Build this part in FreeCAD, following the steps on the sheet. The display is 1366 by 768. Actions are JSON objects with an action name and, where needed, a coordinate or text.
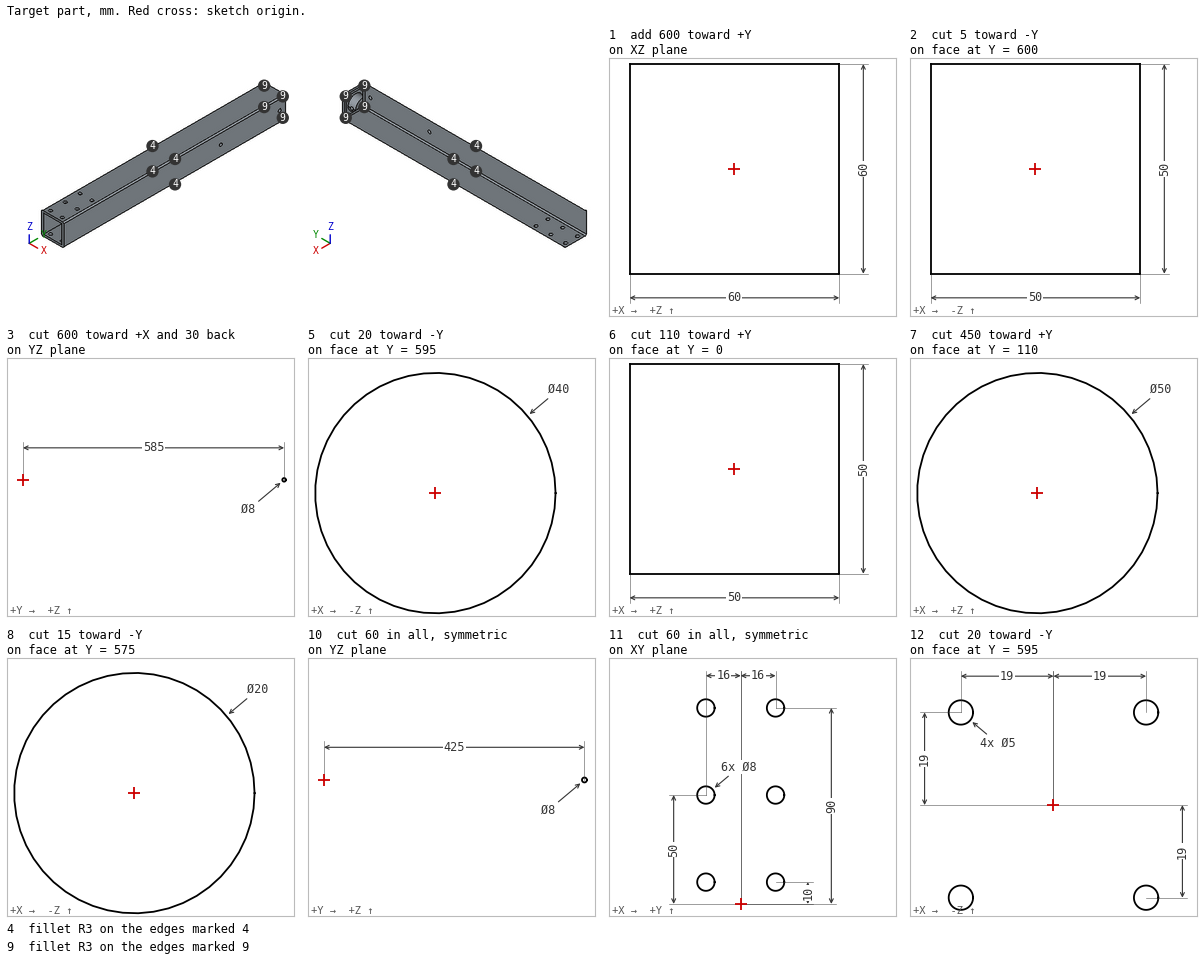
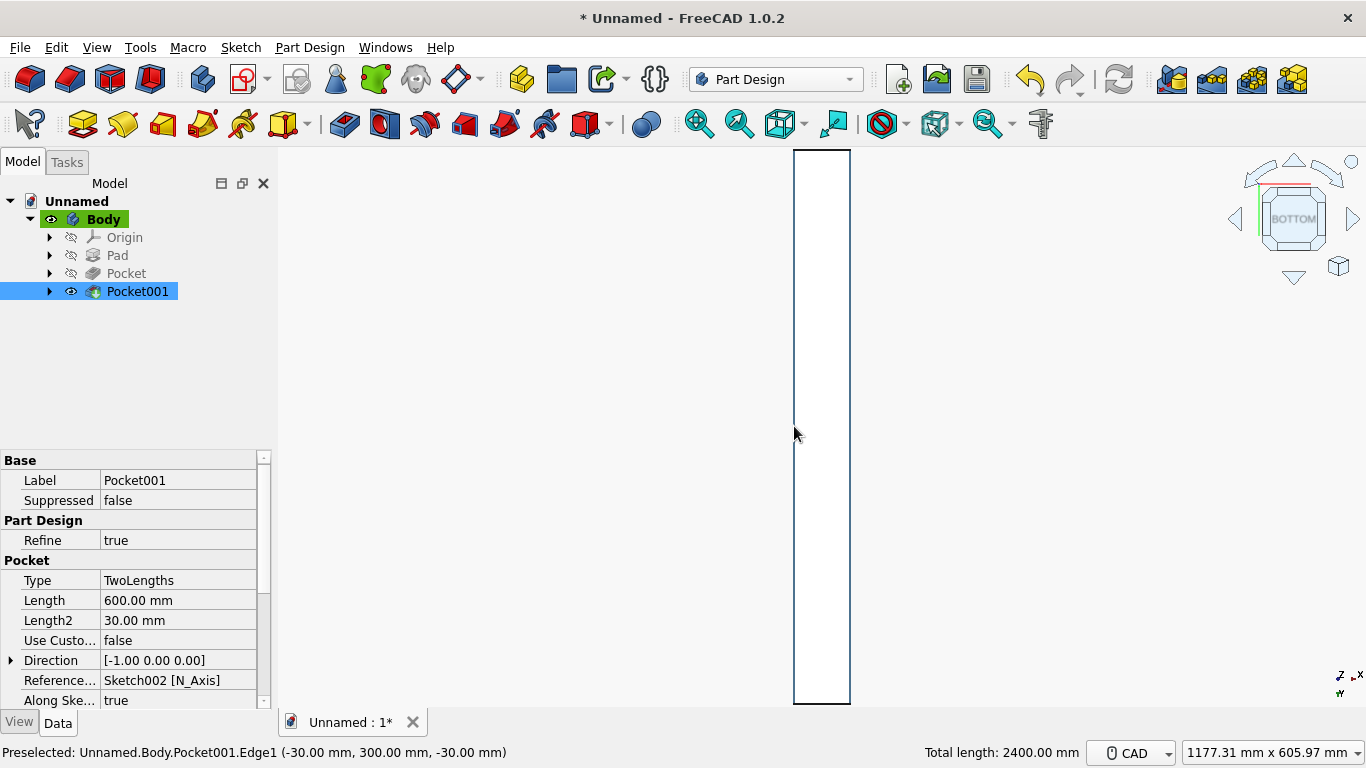
{"action": "left_click", "coordinate": [30, 80]}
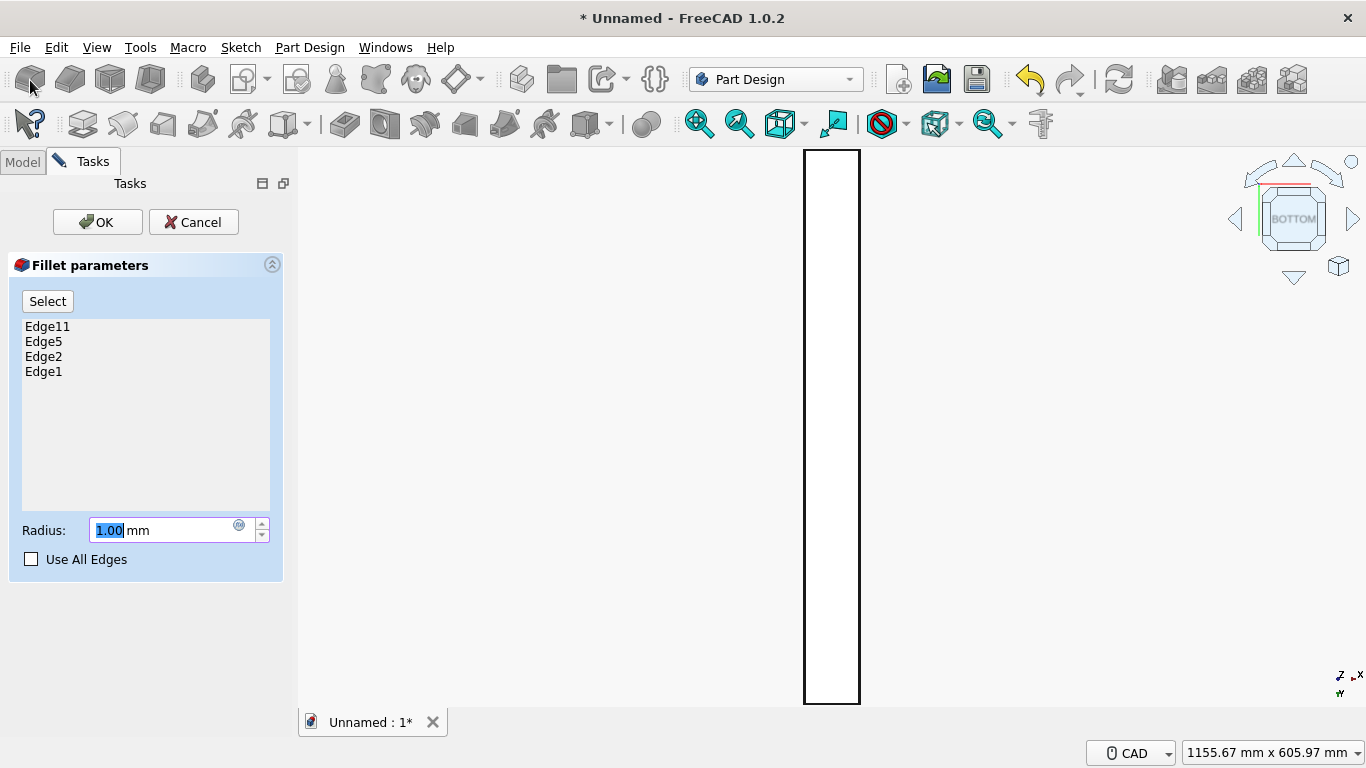
{"action": "type", "text": "3"}
{"action": "key", "text": "Tab"}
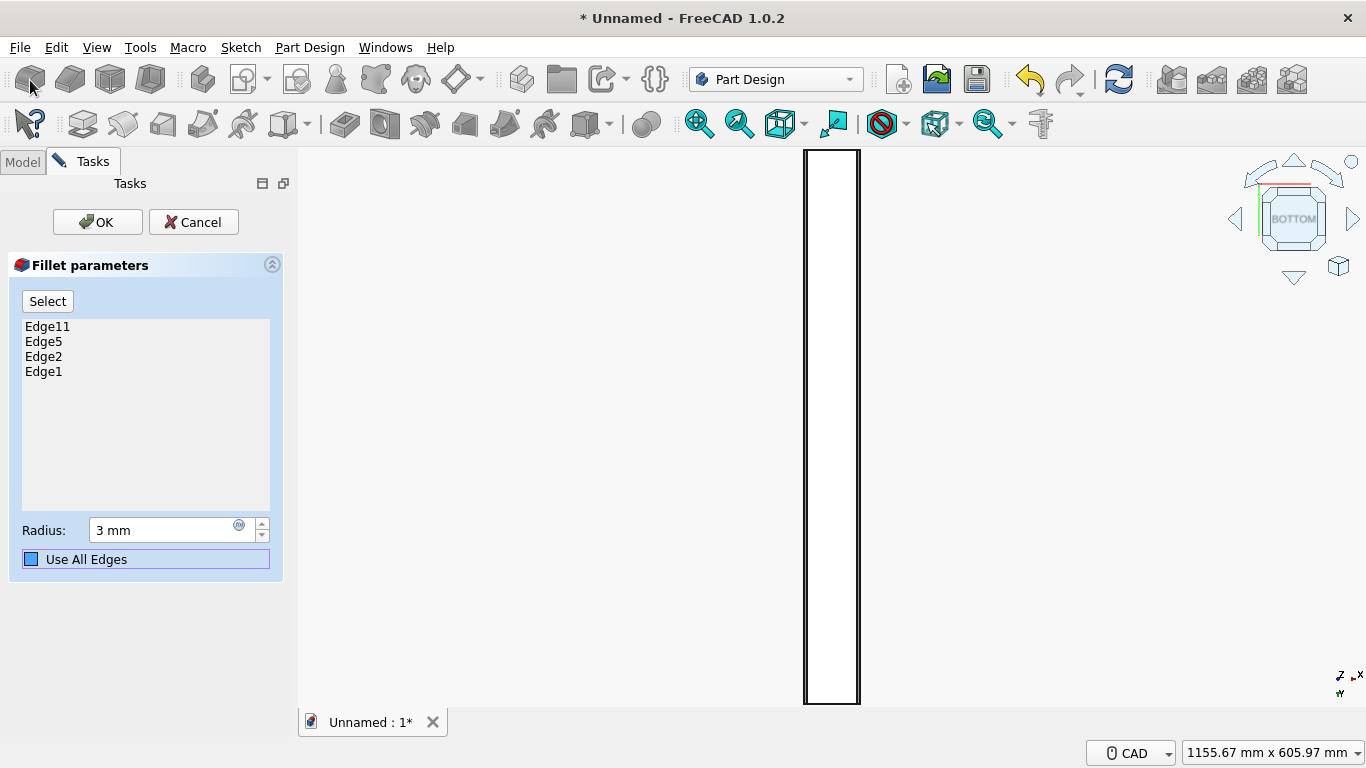
{"action": "left_click", "coordinate": [98, 222]}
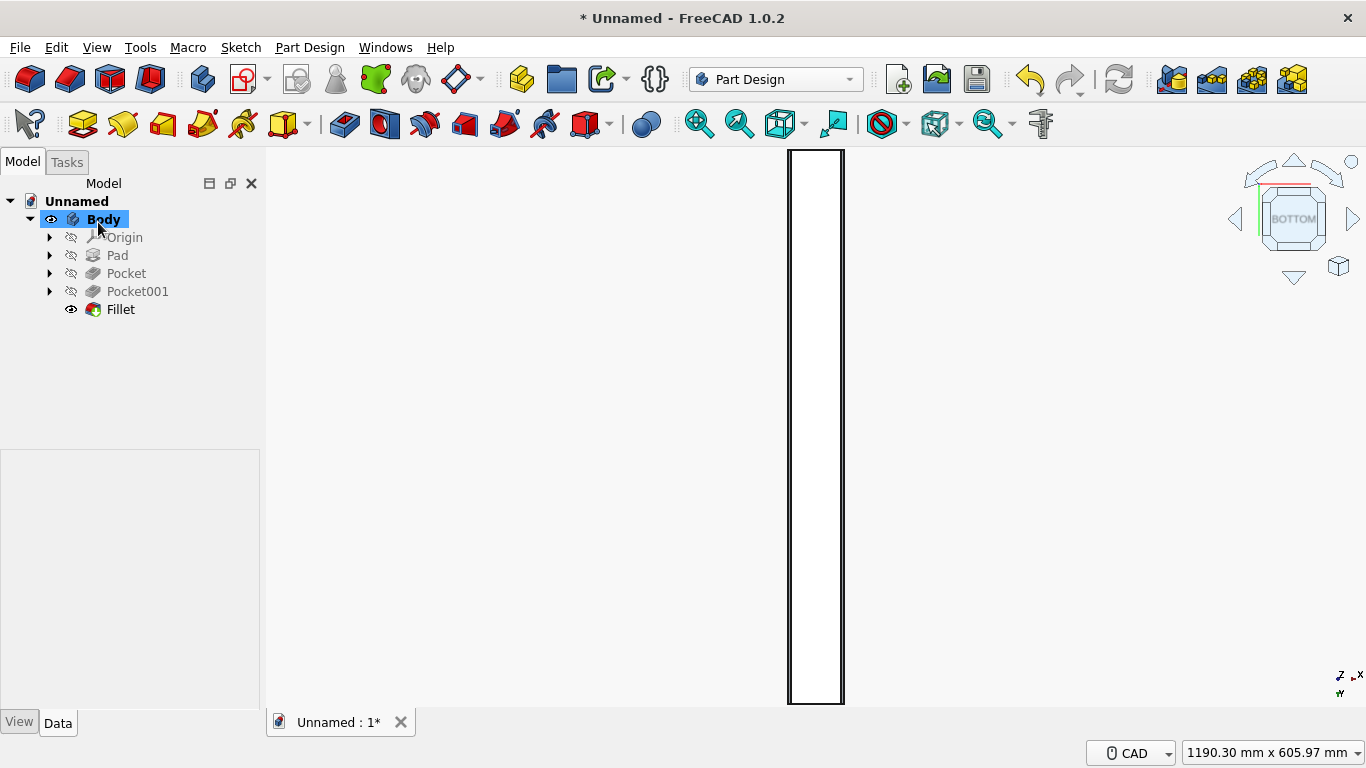
{"action": "key", "text": "4"}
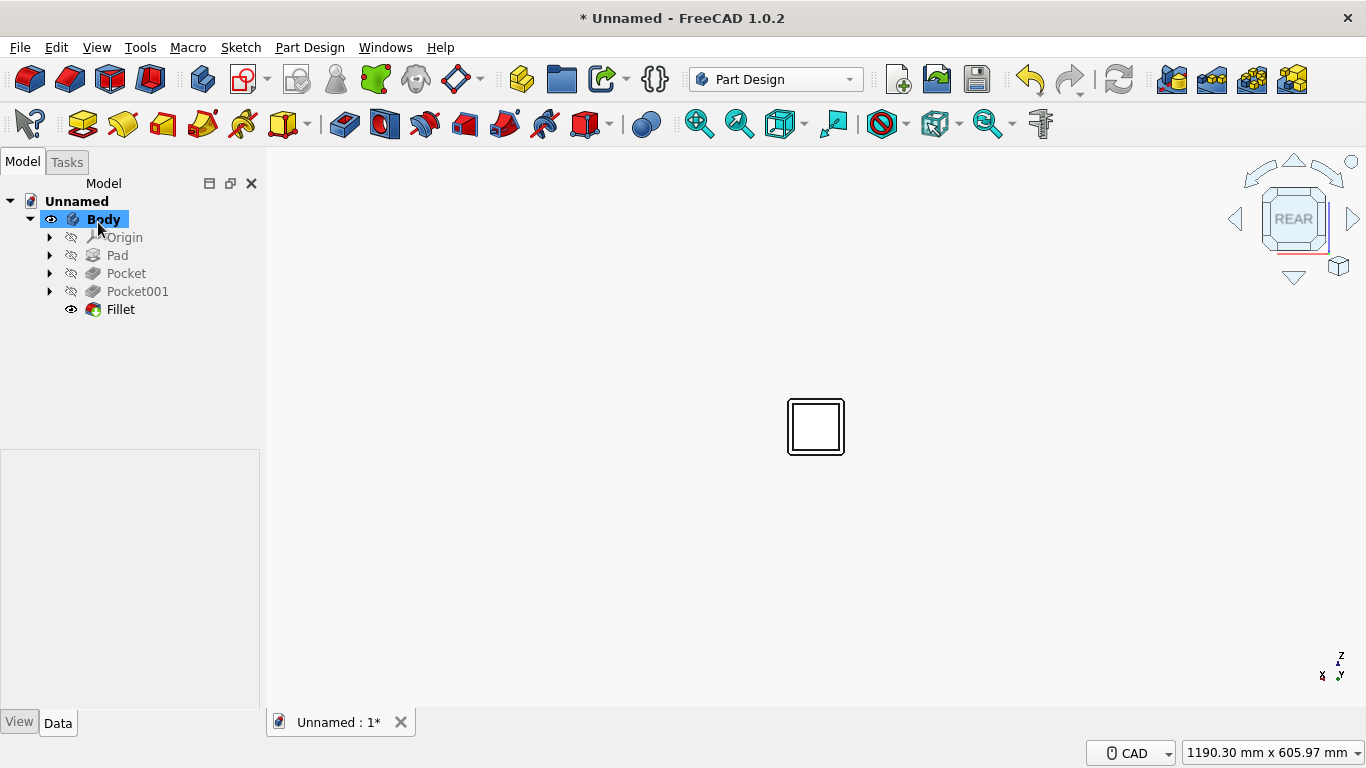
{"action": "left_click", "coordinate": [700, 124]}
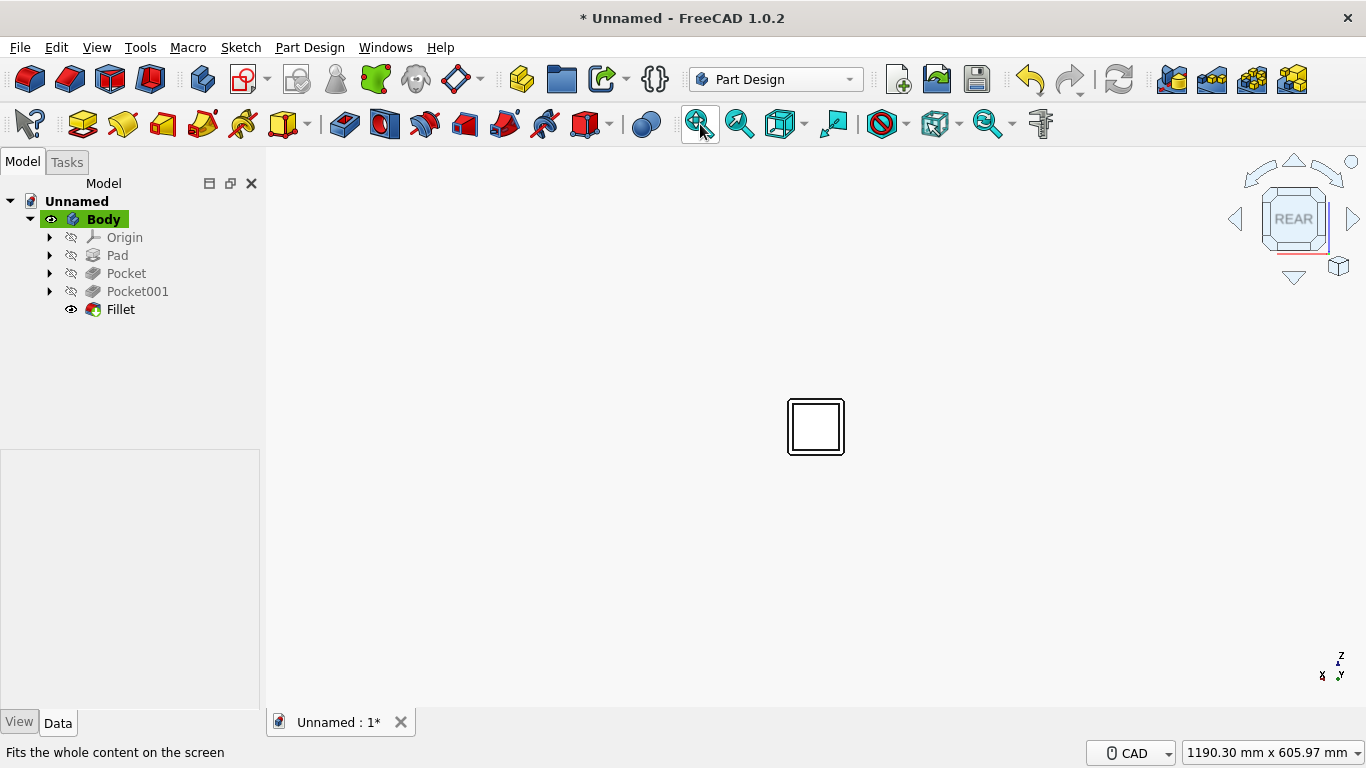
{"action": "left_click", "coordinate": [816, 426]}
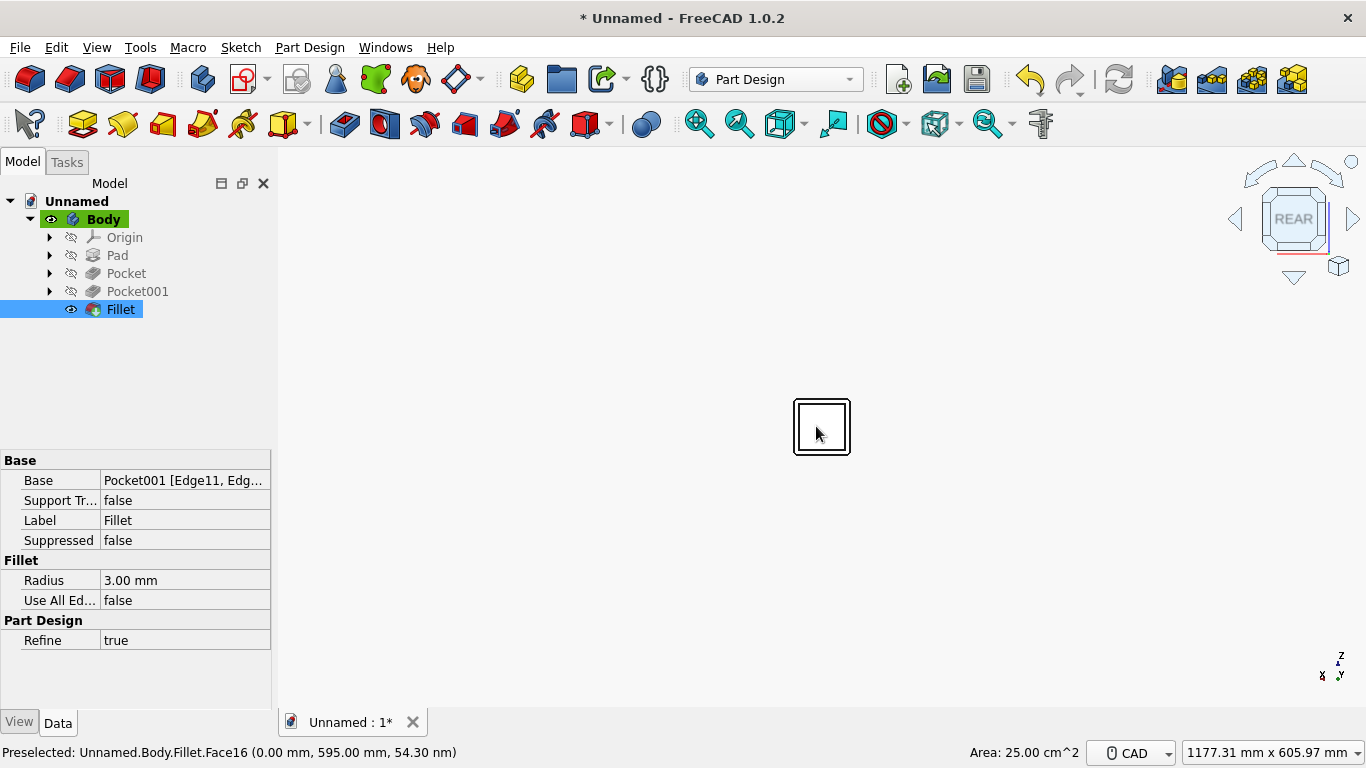
{"action": "left_click", "coordinate": [244, 80]}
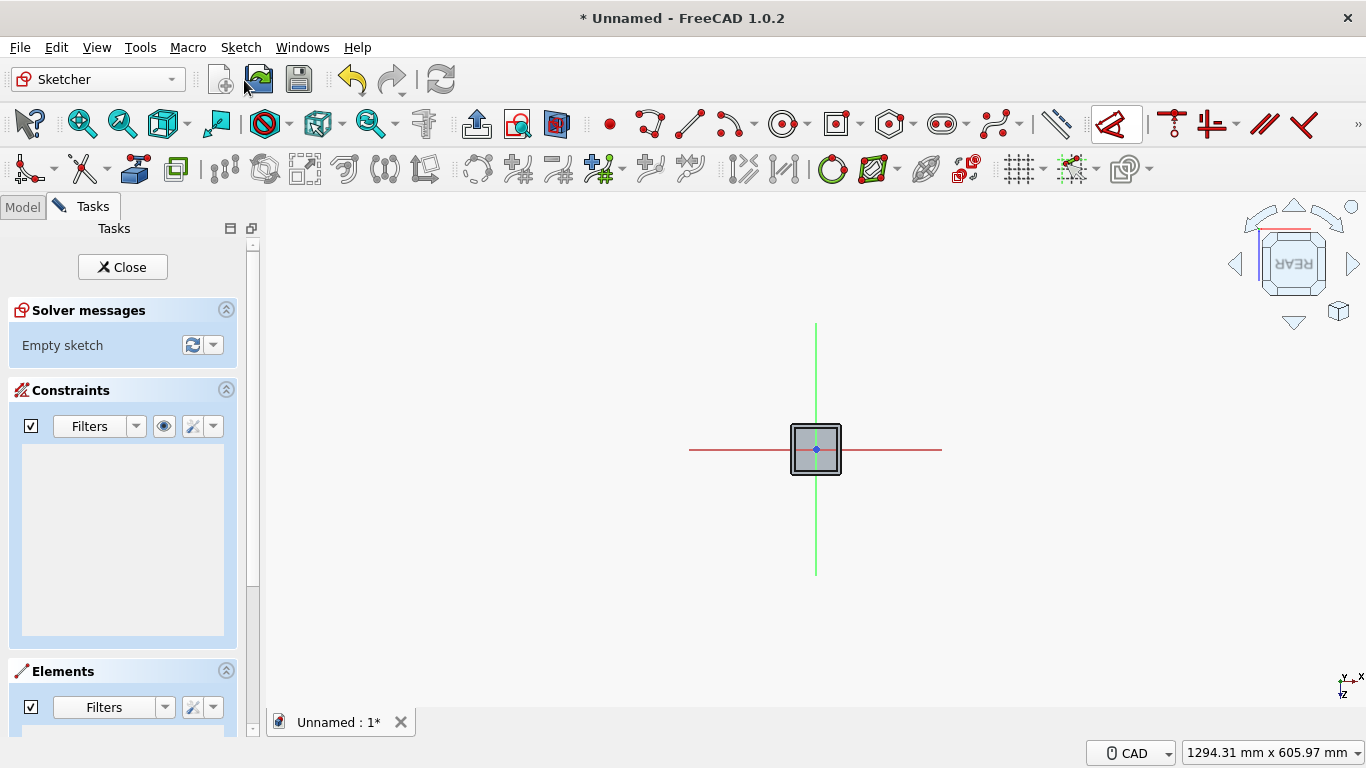
{"action": "scroll", "coordinate": [825, 449], "scroll_direction": "up", "scroll_amount": 11}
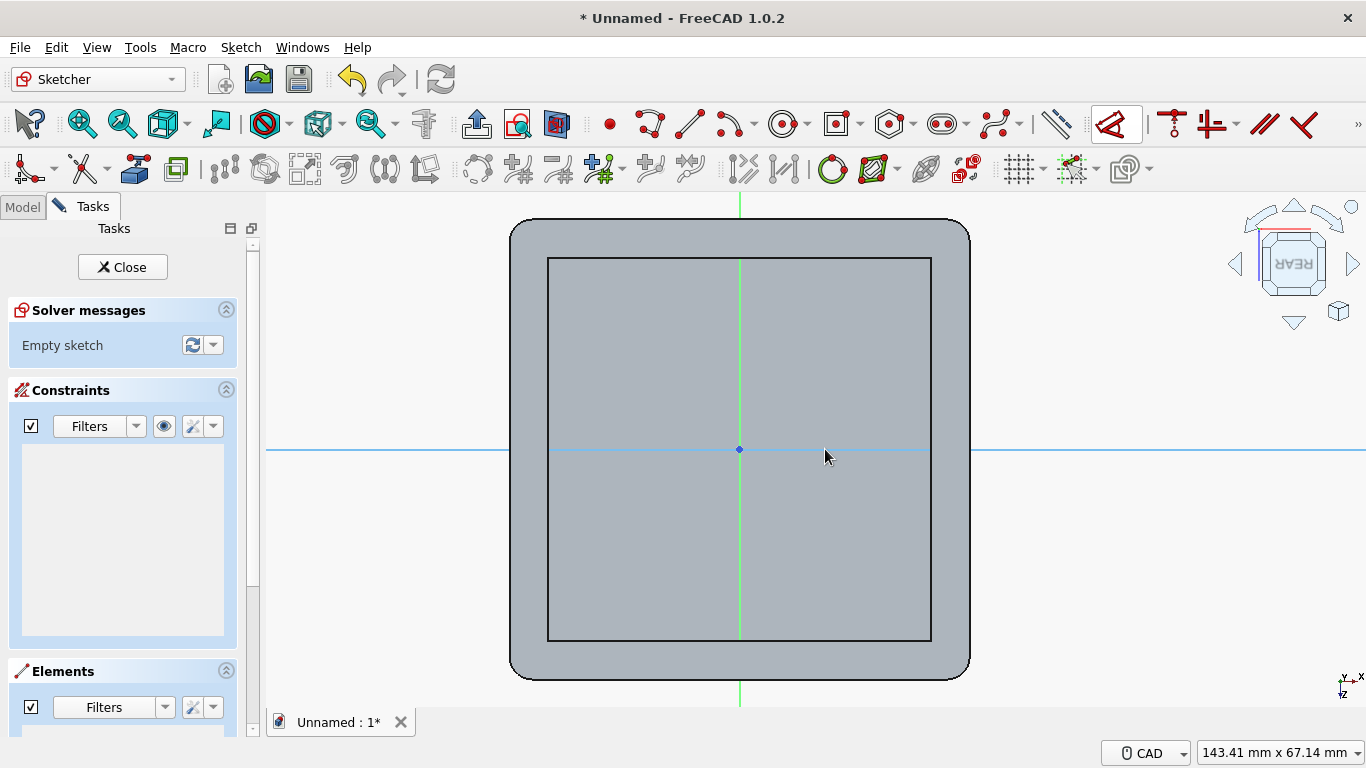
{"action": "left_click", "coordinate": [784, 124]}